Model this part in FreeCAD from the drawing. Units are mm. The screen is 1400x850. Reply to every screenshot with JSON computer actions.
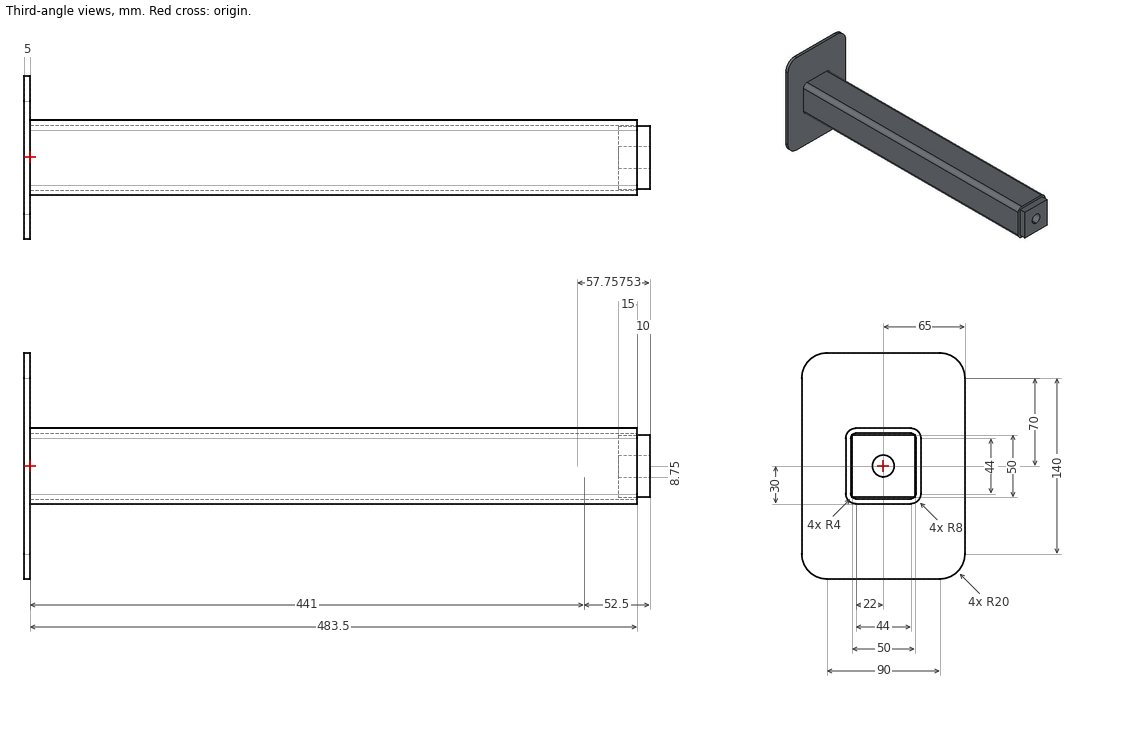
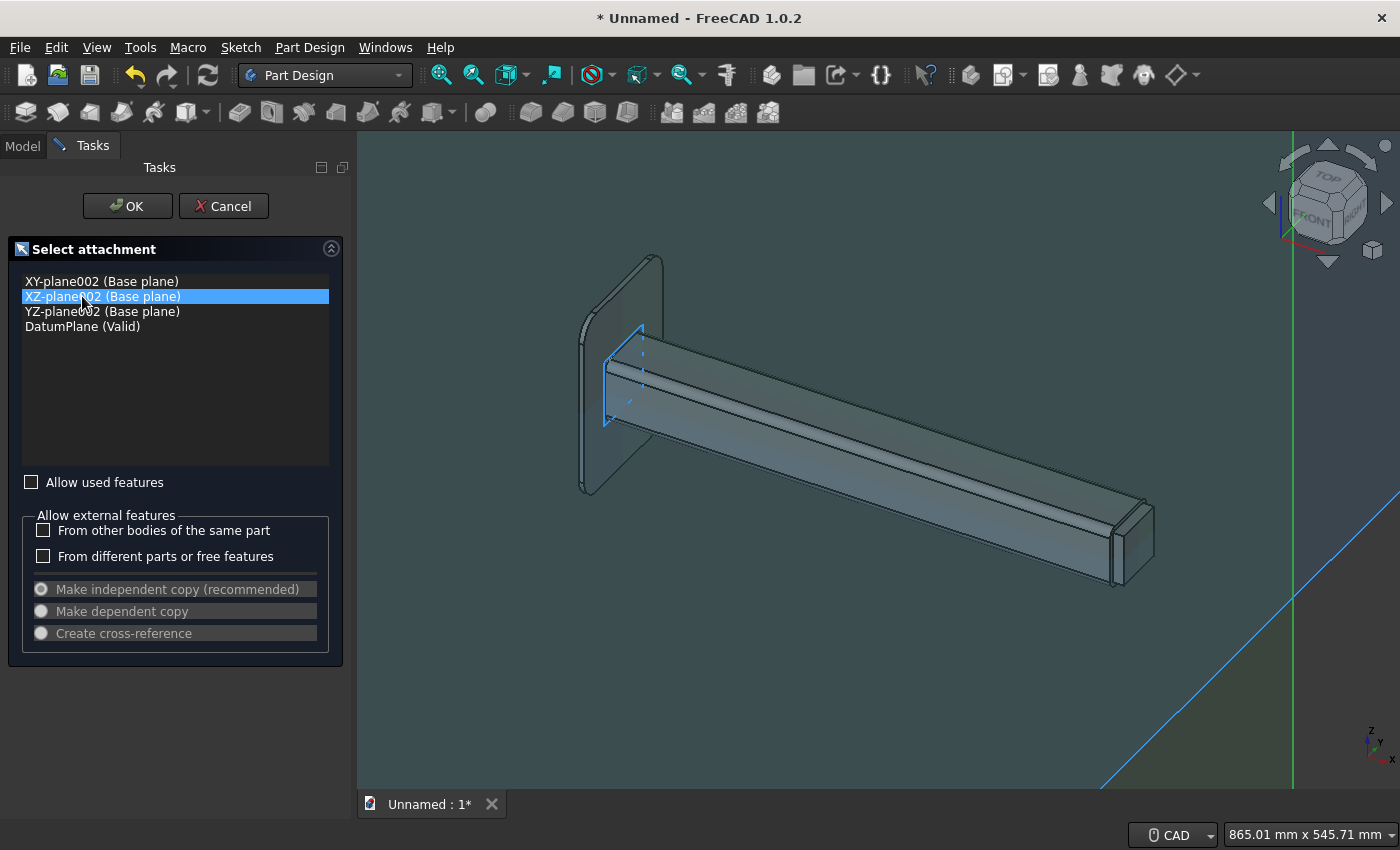
{"action": "left_click", "coordinate": [128, 206]}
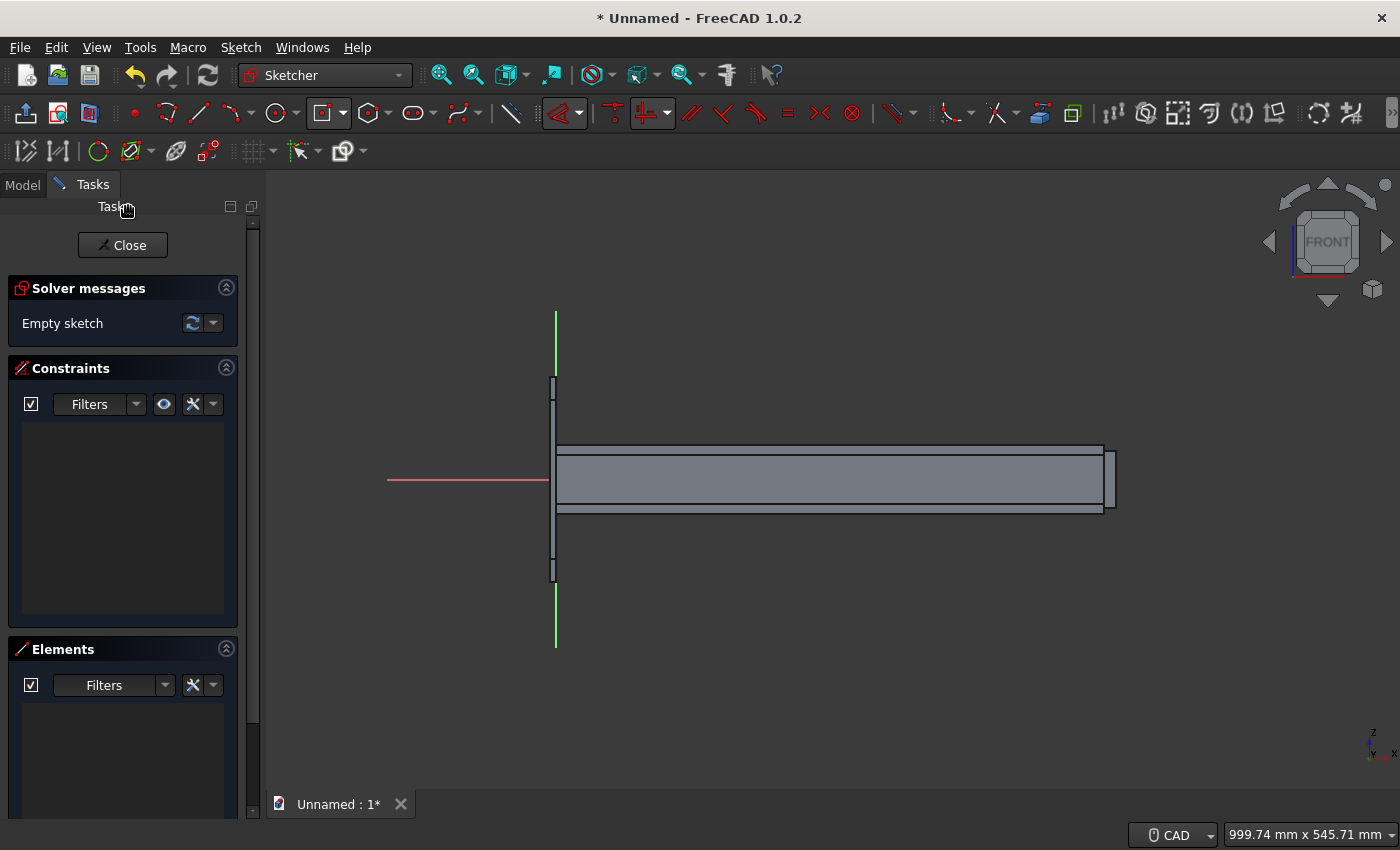
{"action": "key", "text": "q s"}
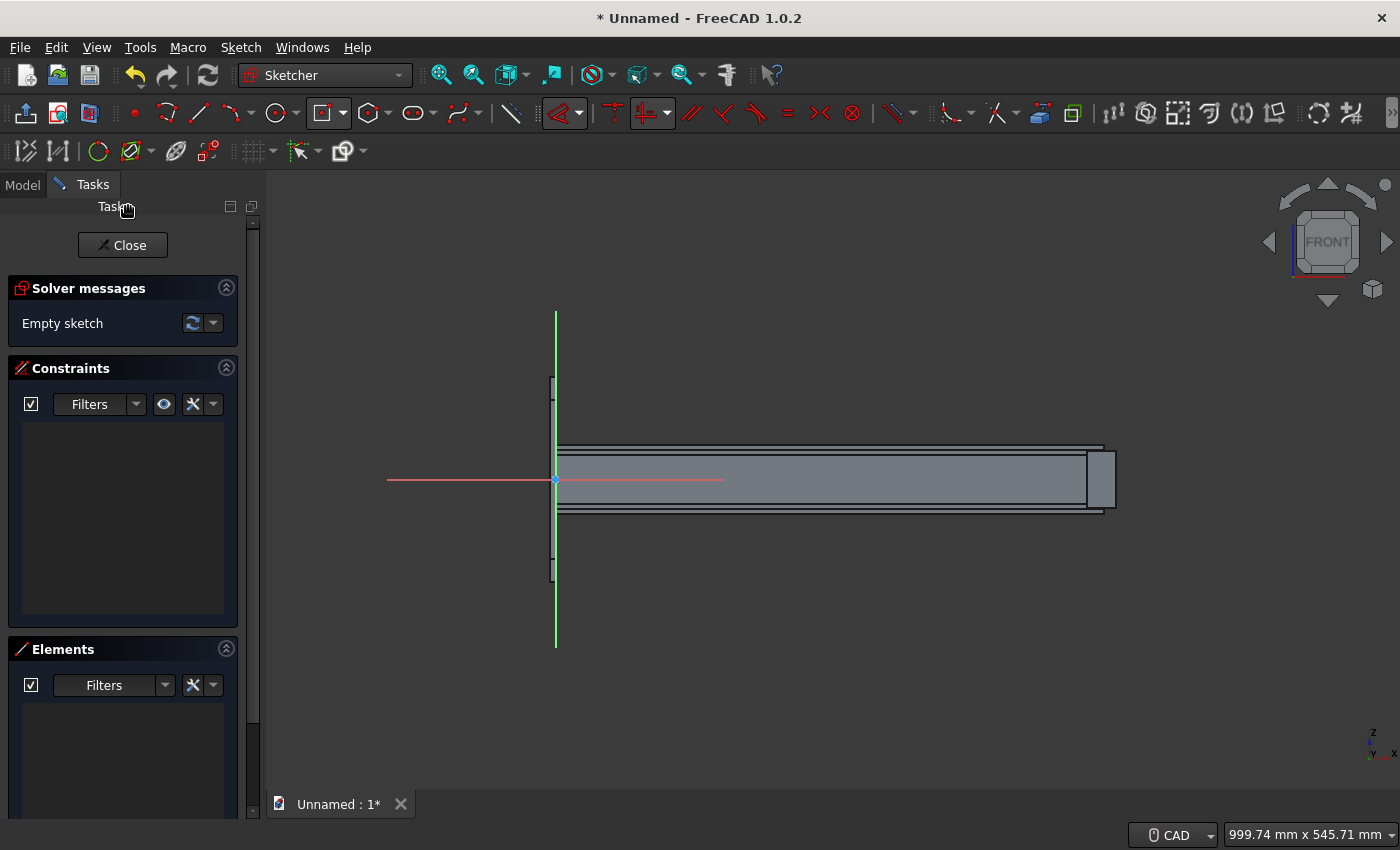
{"action": "scroll", "coordinate": [1115, 485], "scroll_direction": "up", "scroll_amount": 12}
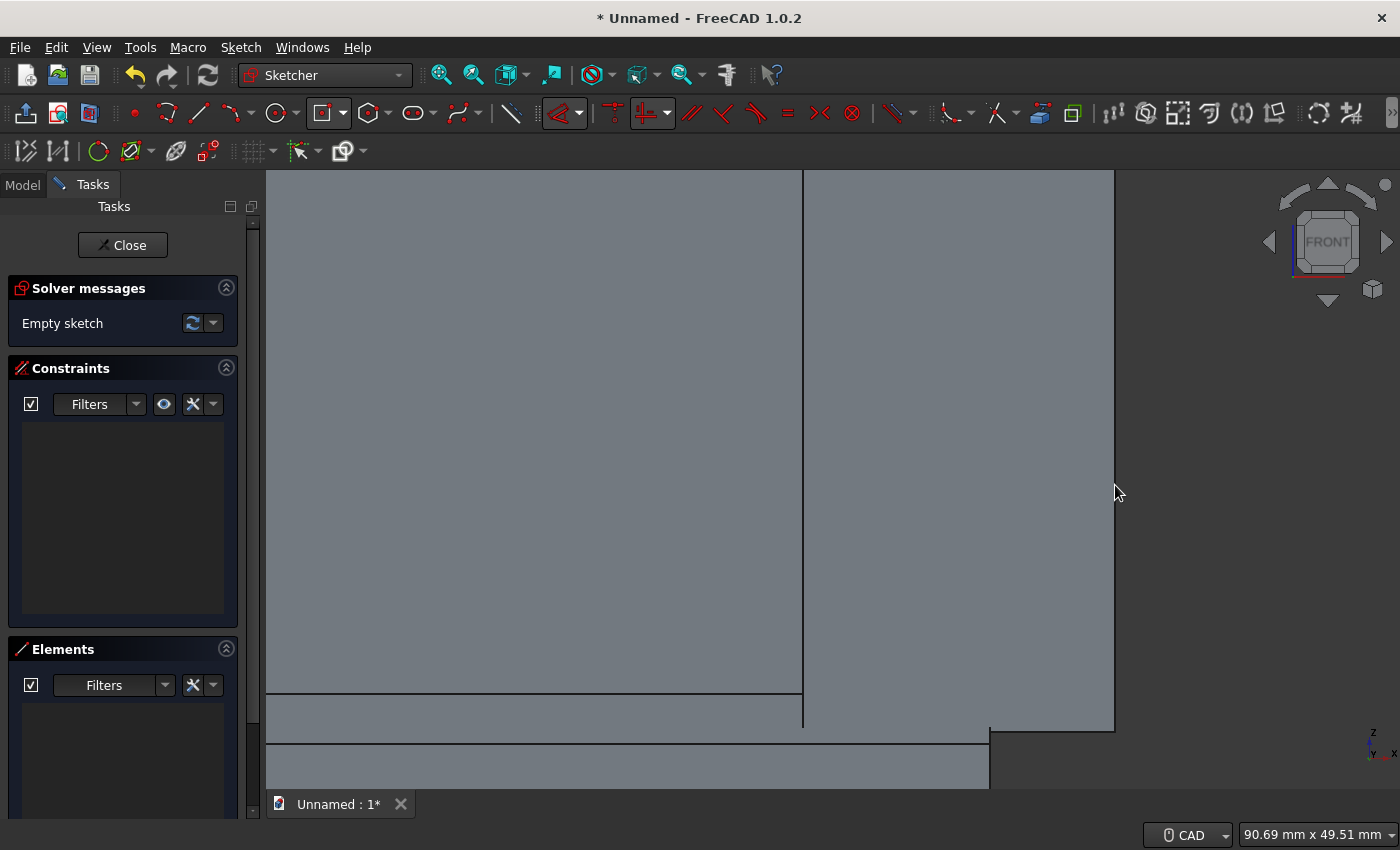
{"action": "left_click", "coordinate": [168, 114]}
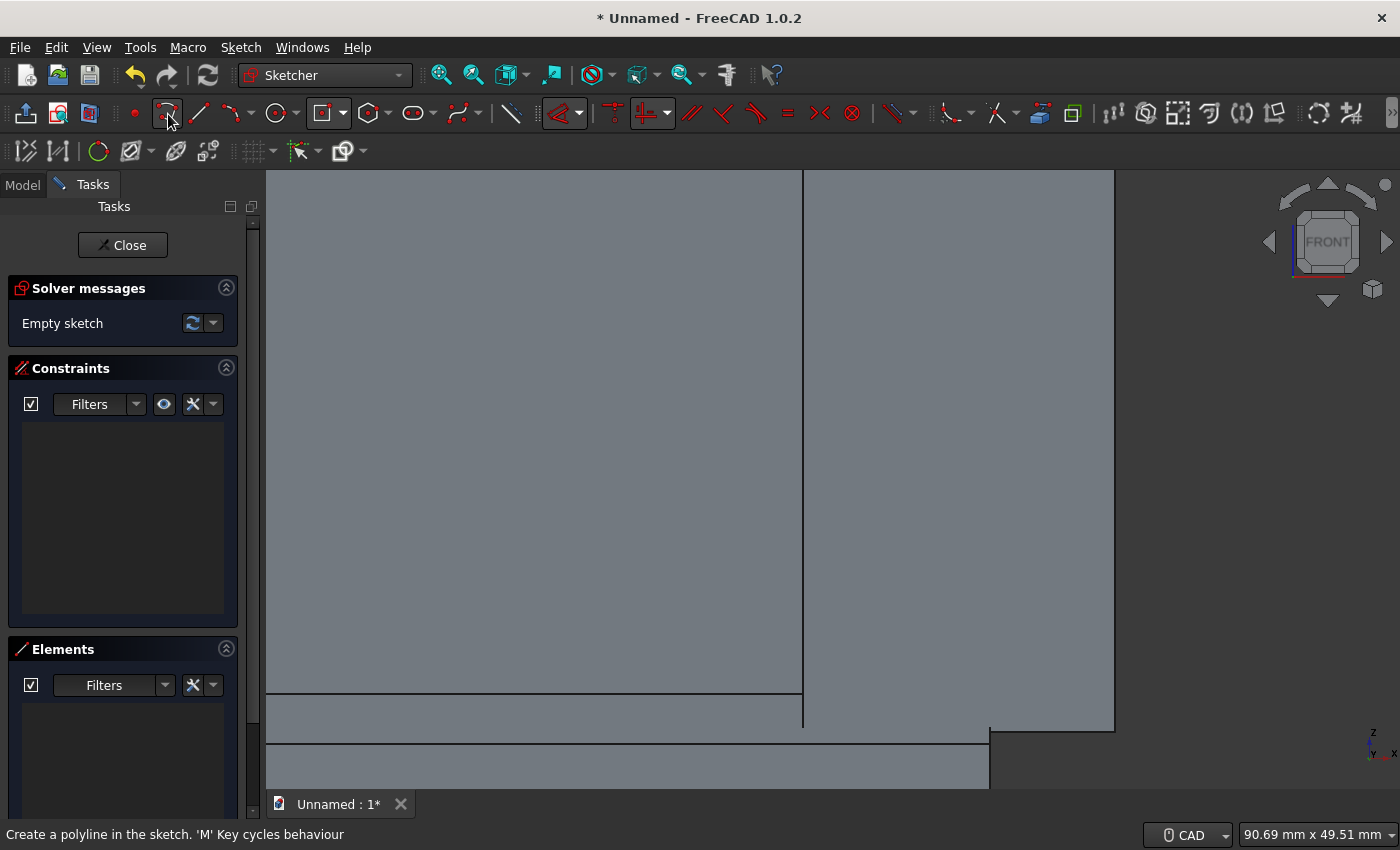
{"action": "left_click", "coordinate": [393, 419]}
{"action": "left_click", "coordinate": [1115, 428]}
{"action": "left_click", "coordinate": [1115, 529]}
{"action": "left_click", "coordinate": [459, 529]}
{"action": "left_click", "coordinate": [393, 420]}
{"action": "key", "text": "Escape"}
{"action": "key", "text": "Escape"}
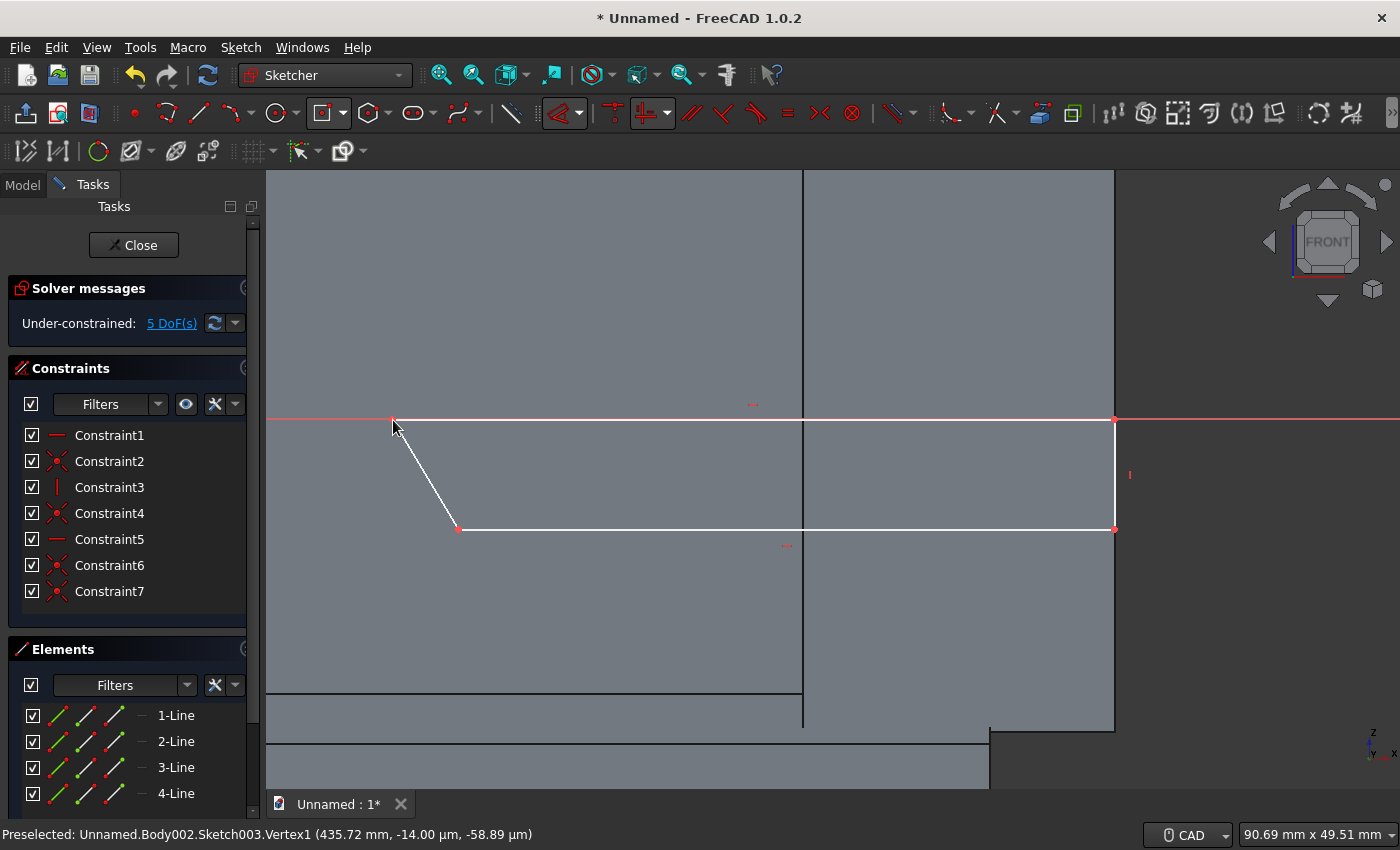
{"action": "left_click", "coordinate": [393, 420]}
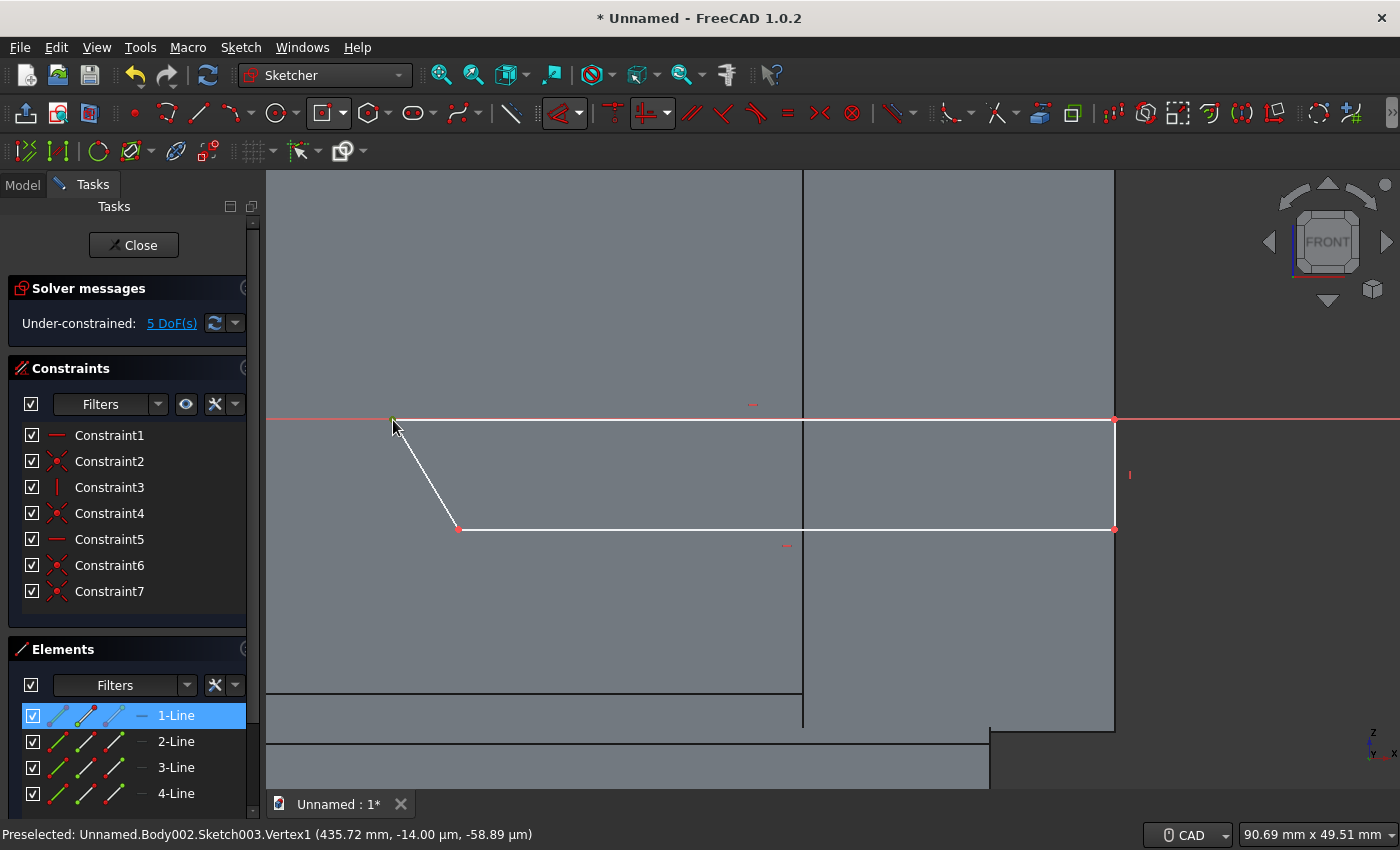
{"action": "left_click", "coordinate": [361, 419]}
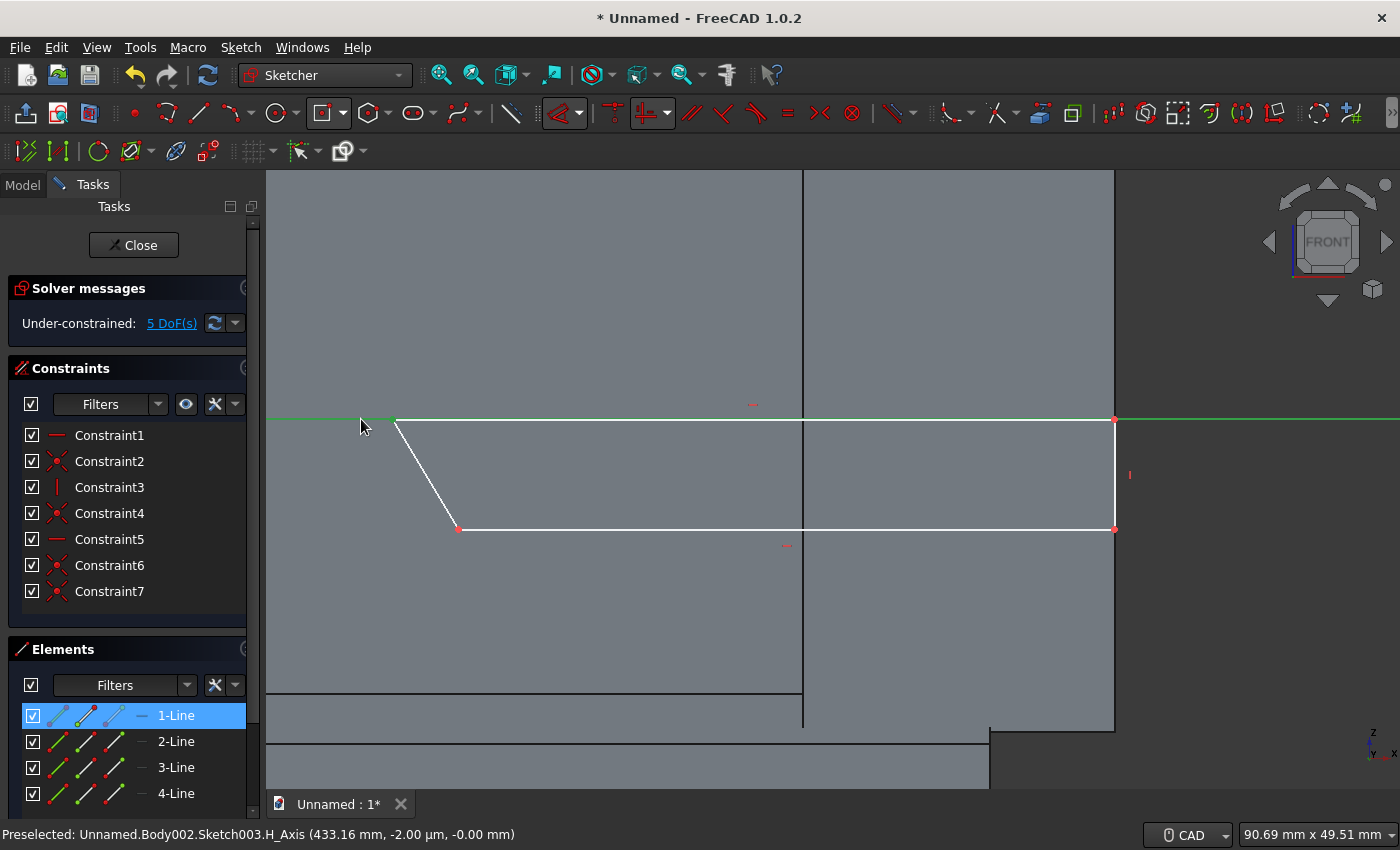
{"action": "key", "text": "c"}